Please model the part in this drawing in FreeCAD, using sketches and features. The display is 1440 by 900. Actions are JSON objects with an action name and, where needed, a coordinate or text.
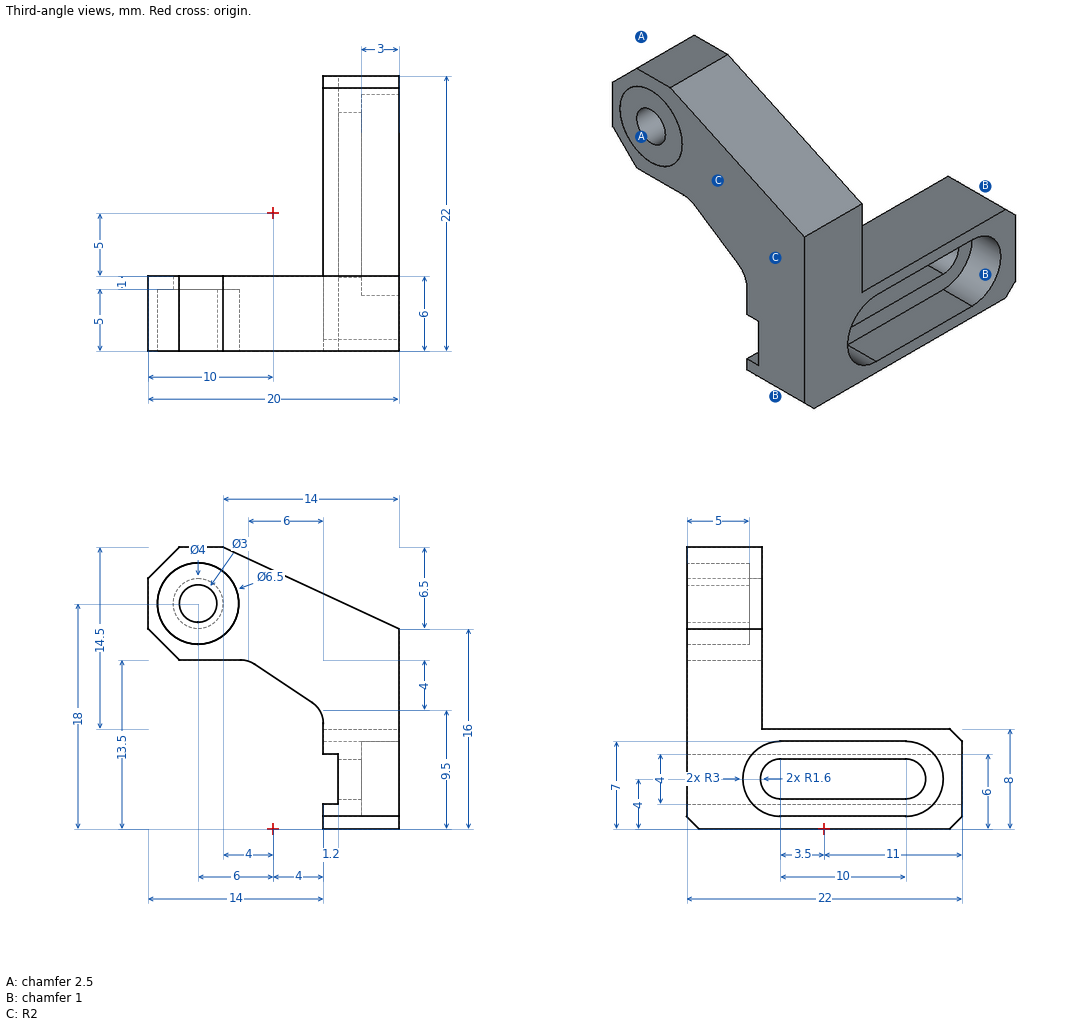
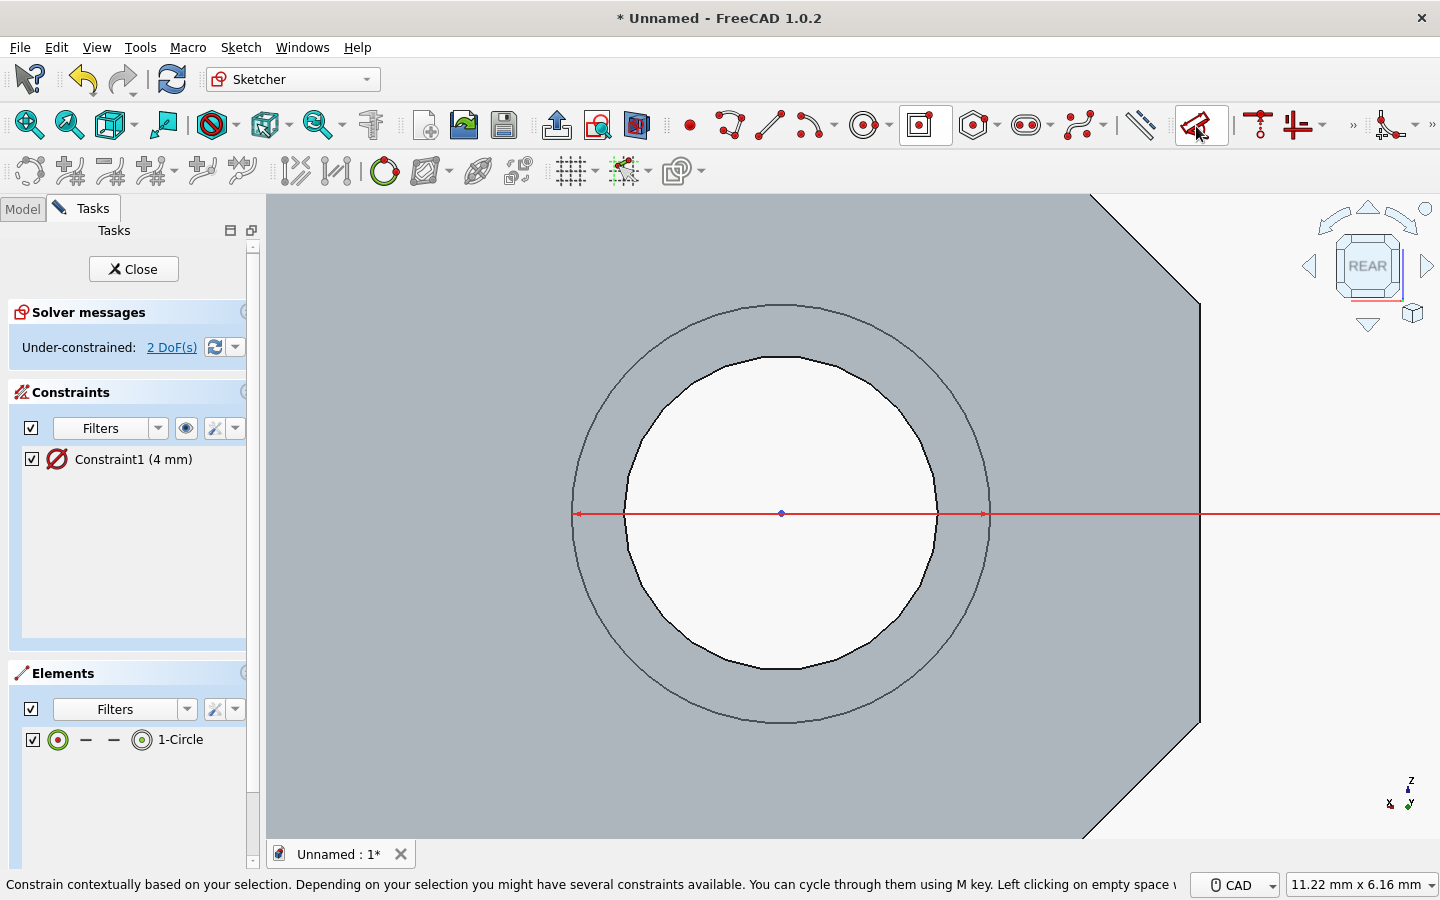
{"action": "left_click", "coordinate": [781, 514]}
{"action": "left_click", "coordinate": [537, 480]}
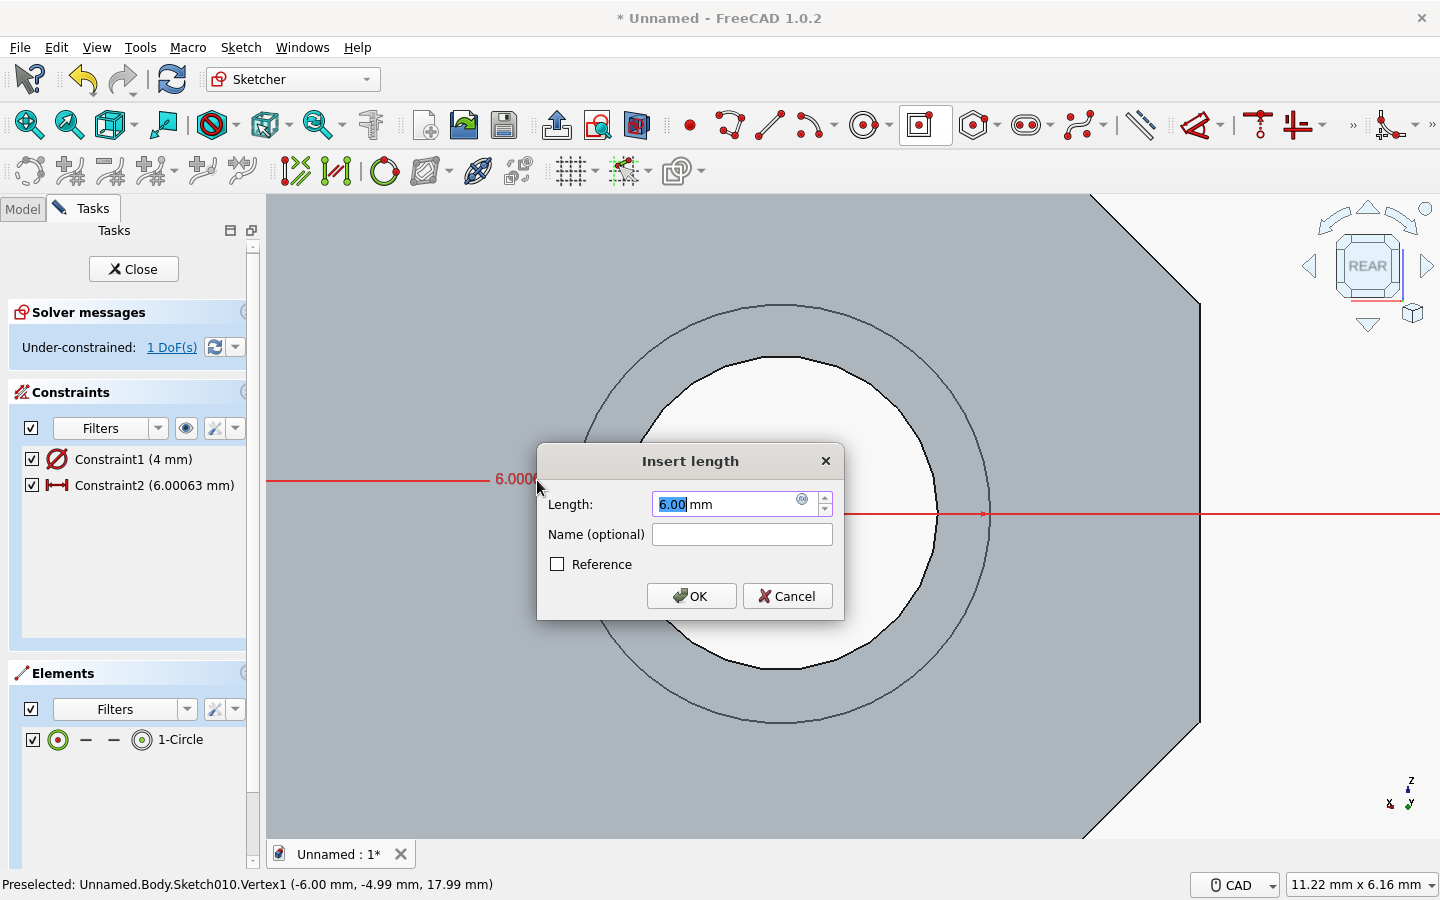
{"action": "type", "text": "6"}
{"action": "key", "text": "Return"}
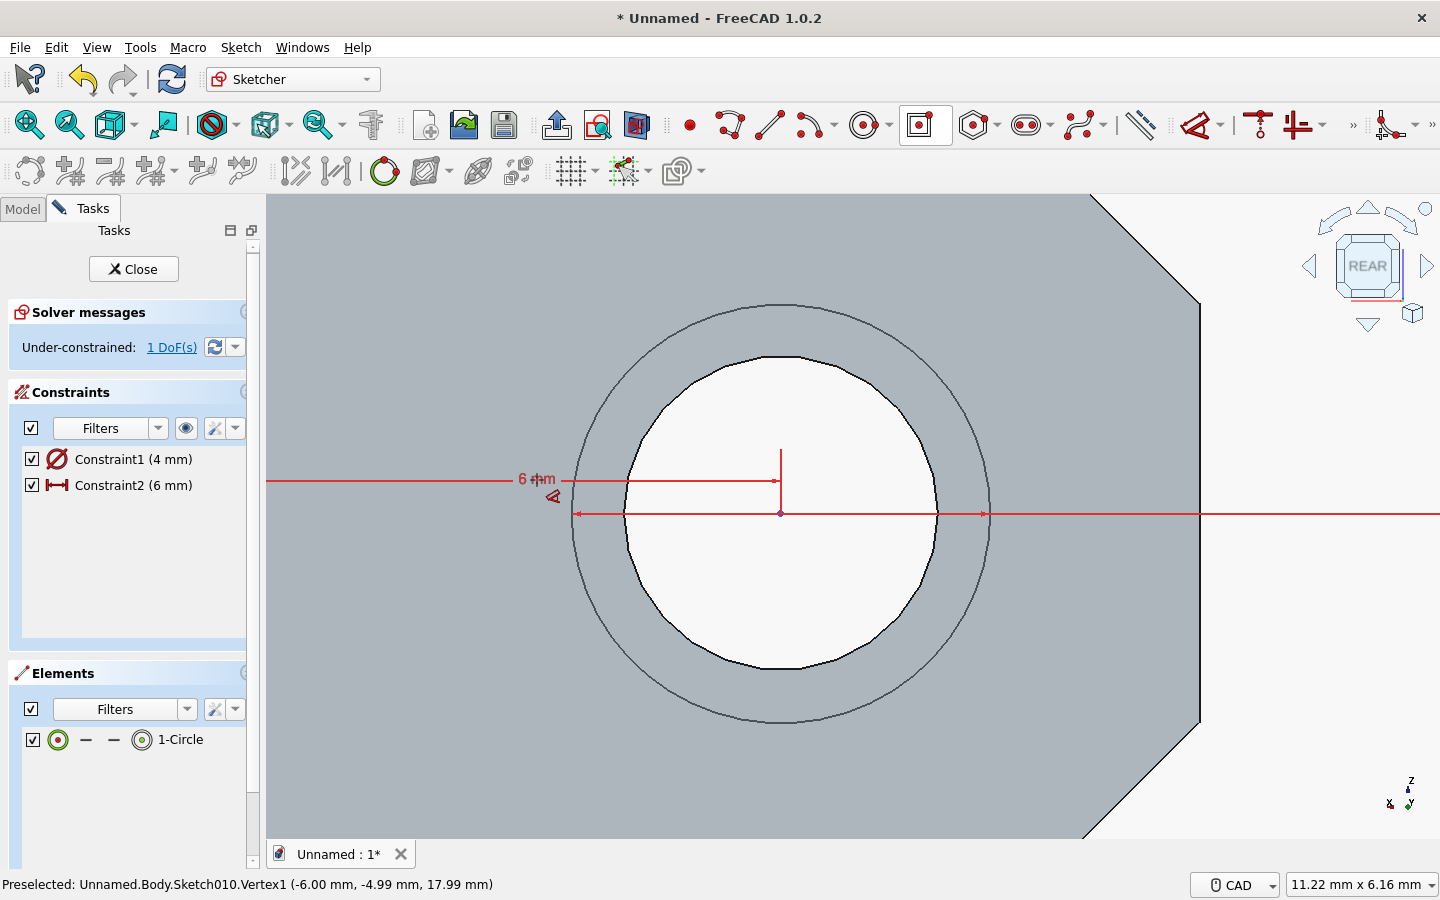
{"action": "left_click", "coordinate": [781, 514]}
{"action": "left_click", "coordinate": [815, 662]}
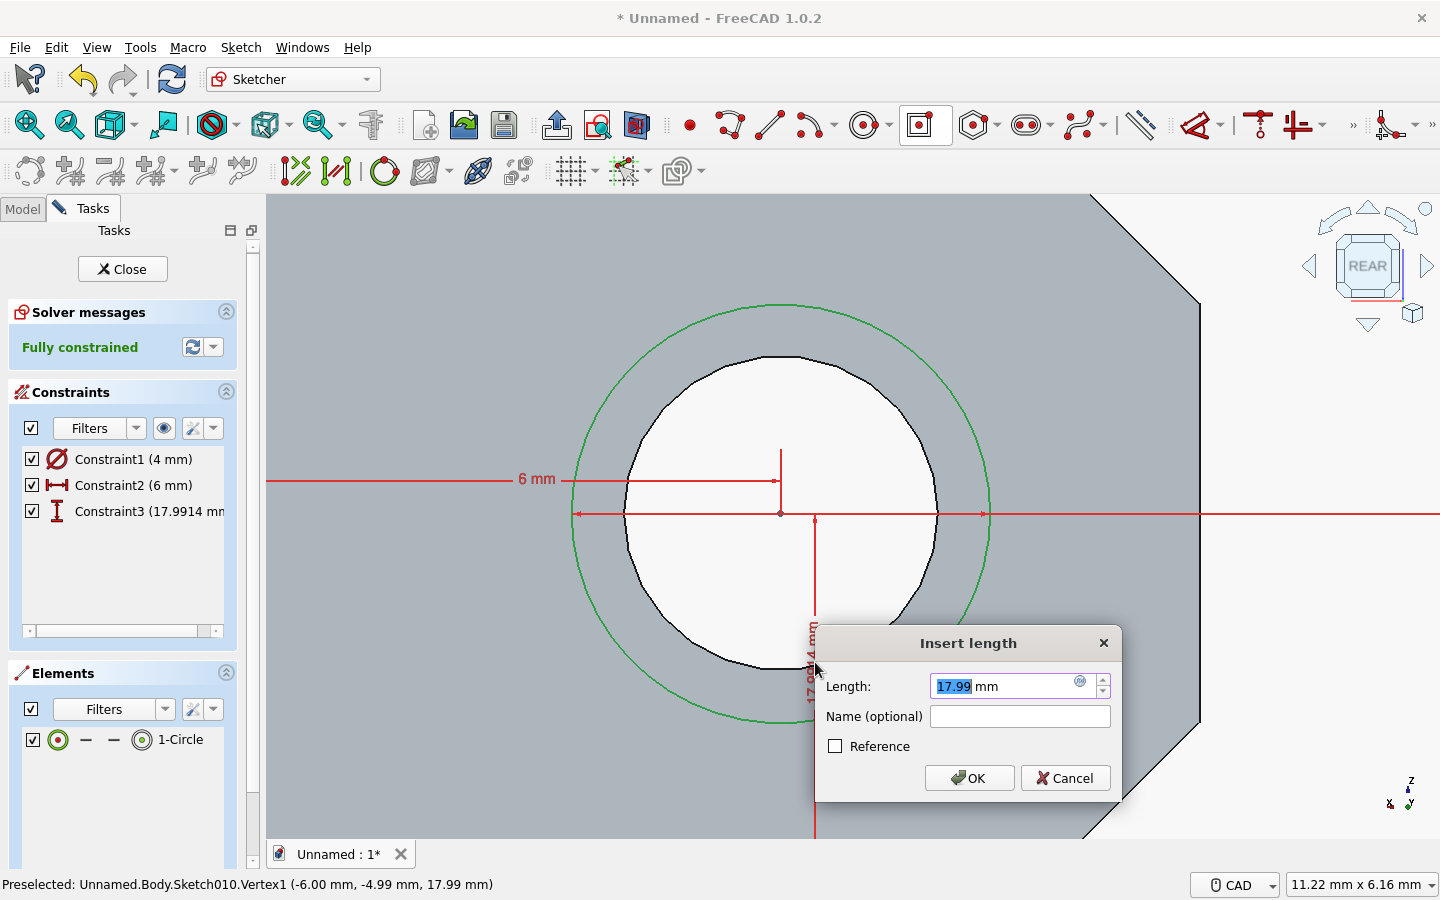
{"action": "type", "text": "18"}
{"action": "key", "text": "Return"}
{"action": "key", "text": "Escape"}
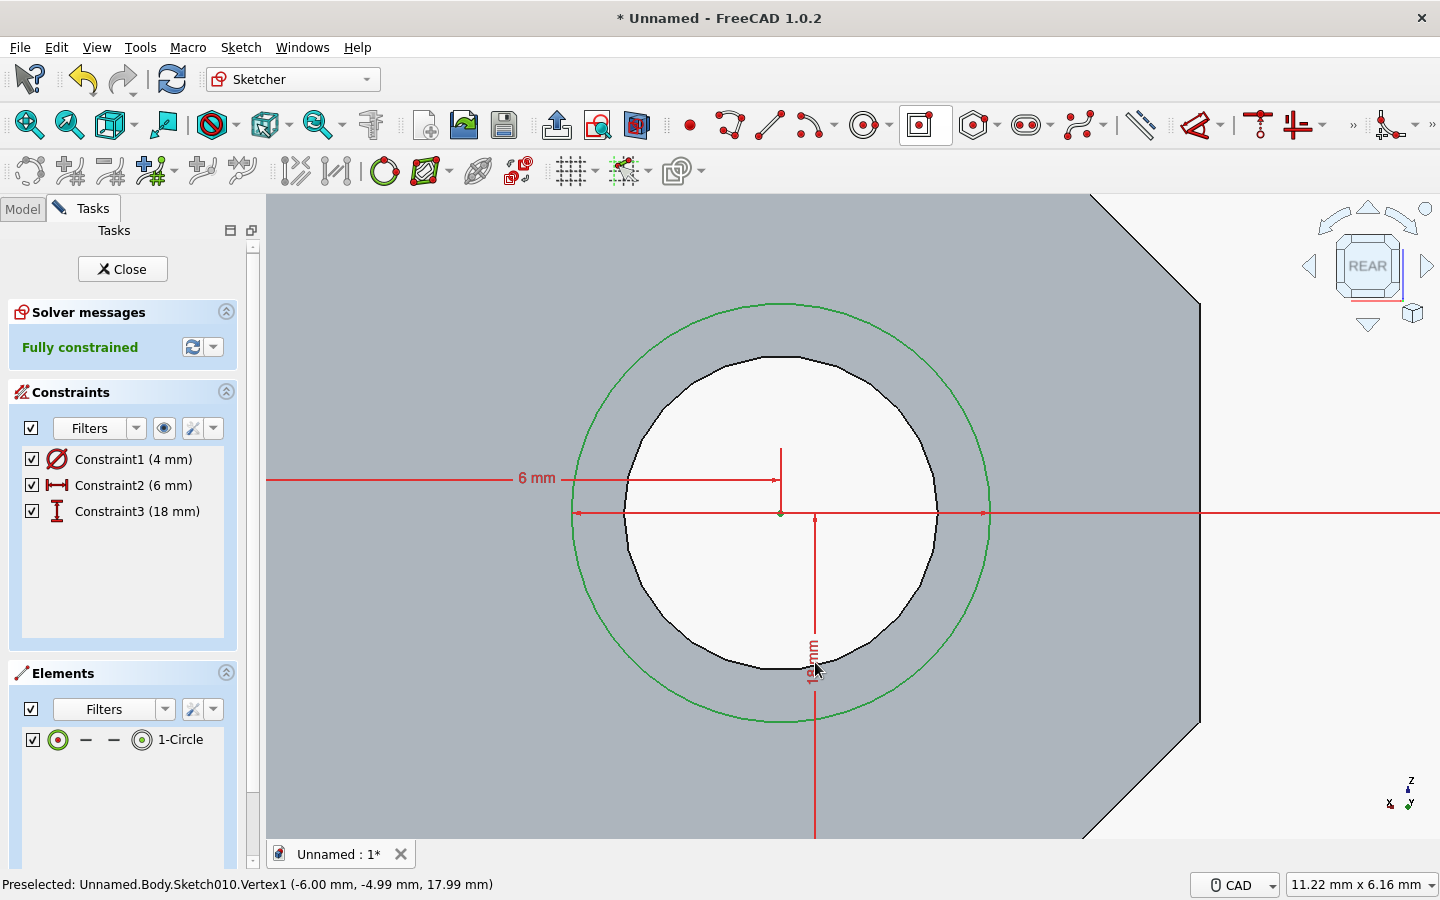
{"action": "left_click", "coordinate": [123, 269]}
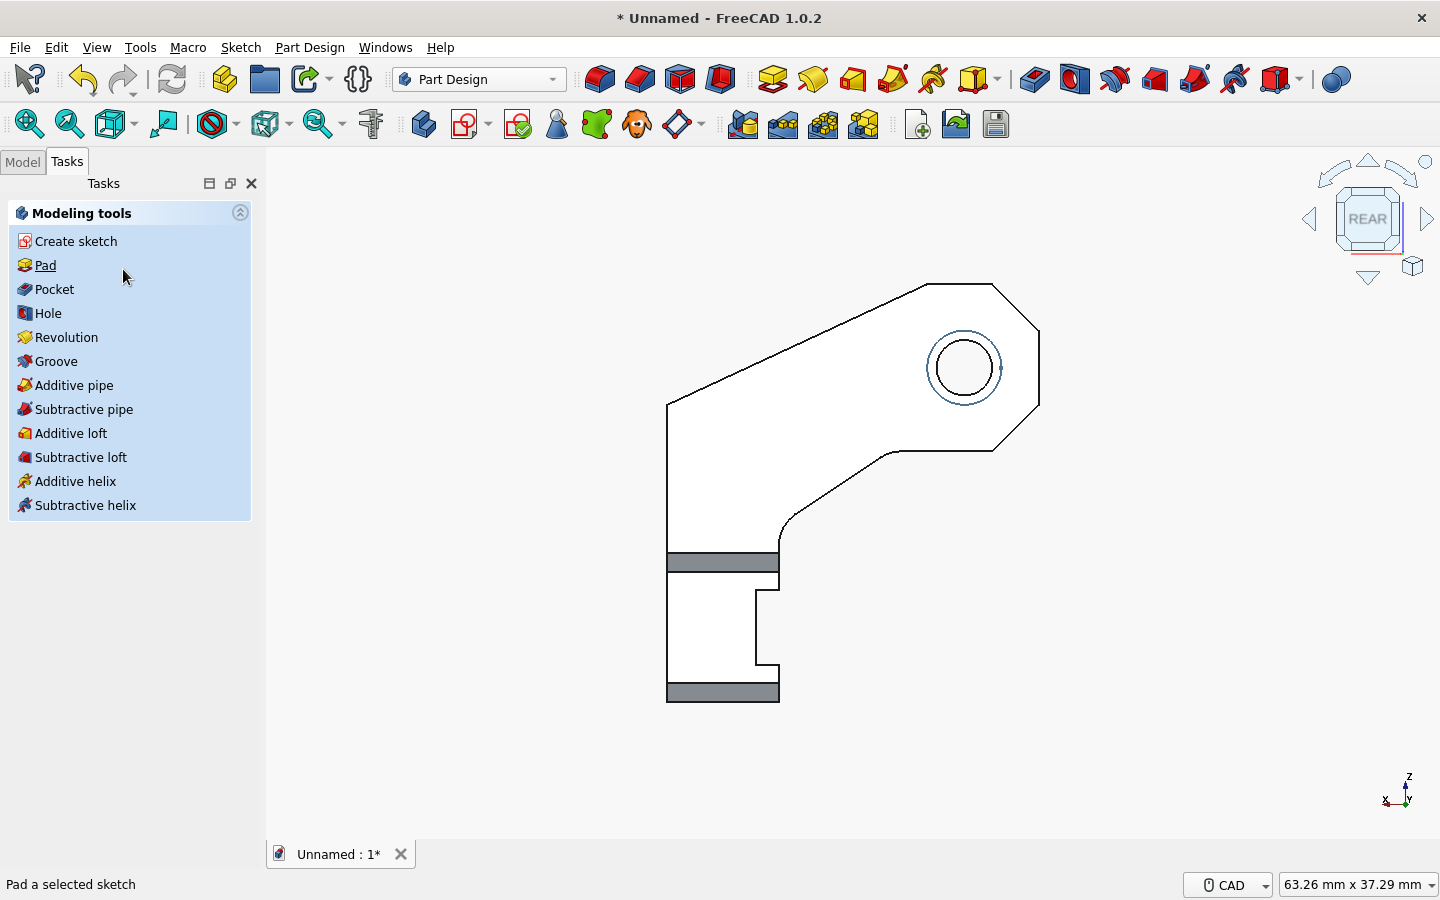
{"action": "left_click", "coordinate": [1036, 80]}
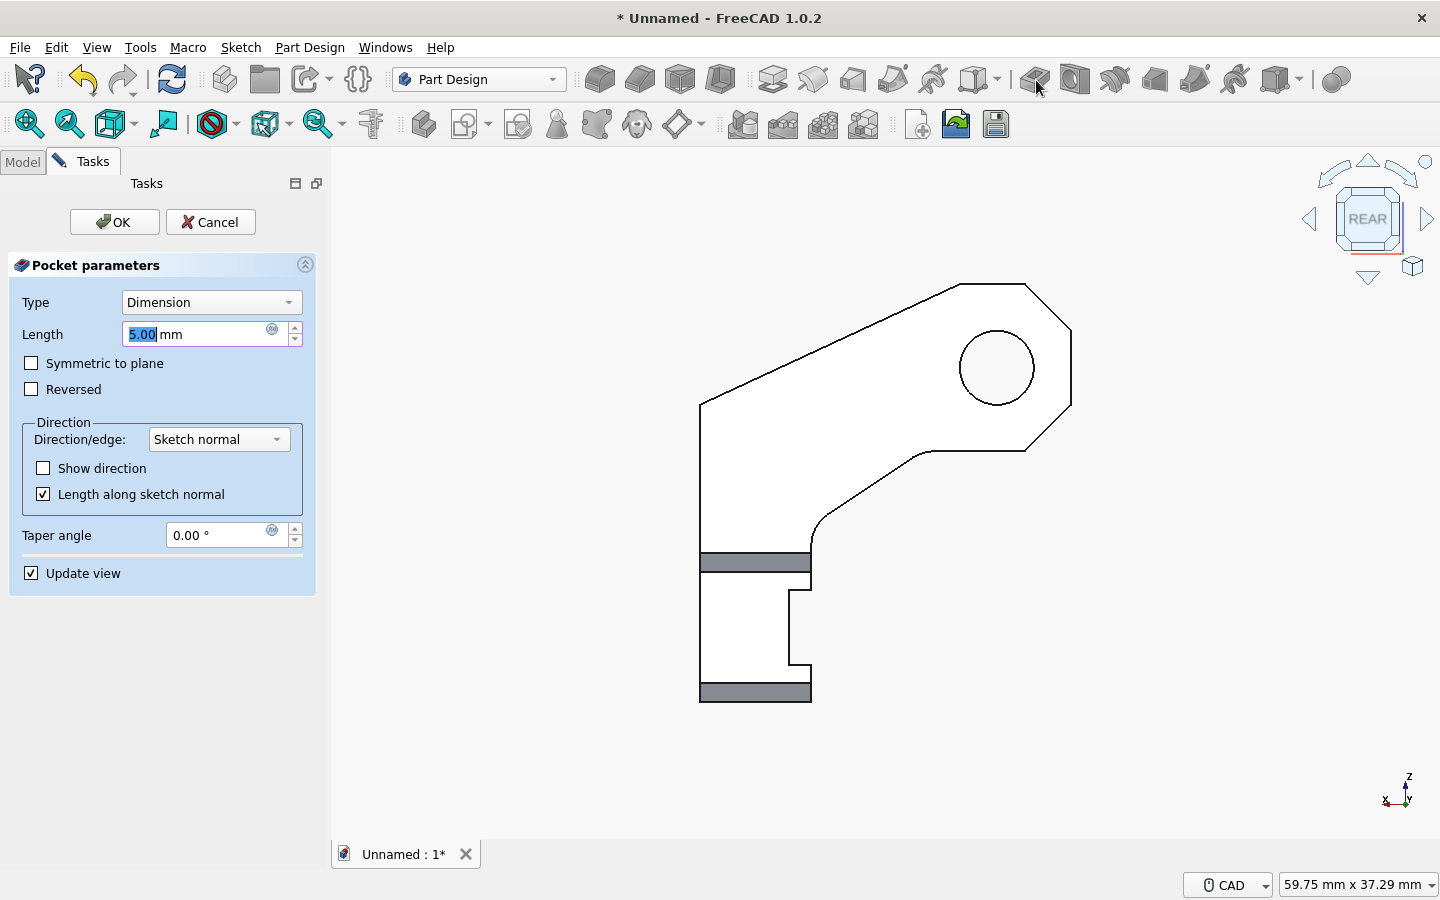
{"action": "type", "text": "1"}
{"action": "key", "text": "Tab"}